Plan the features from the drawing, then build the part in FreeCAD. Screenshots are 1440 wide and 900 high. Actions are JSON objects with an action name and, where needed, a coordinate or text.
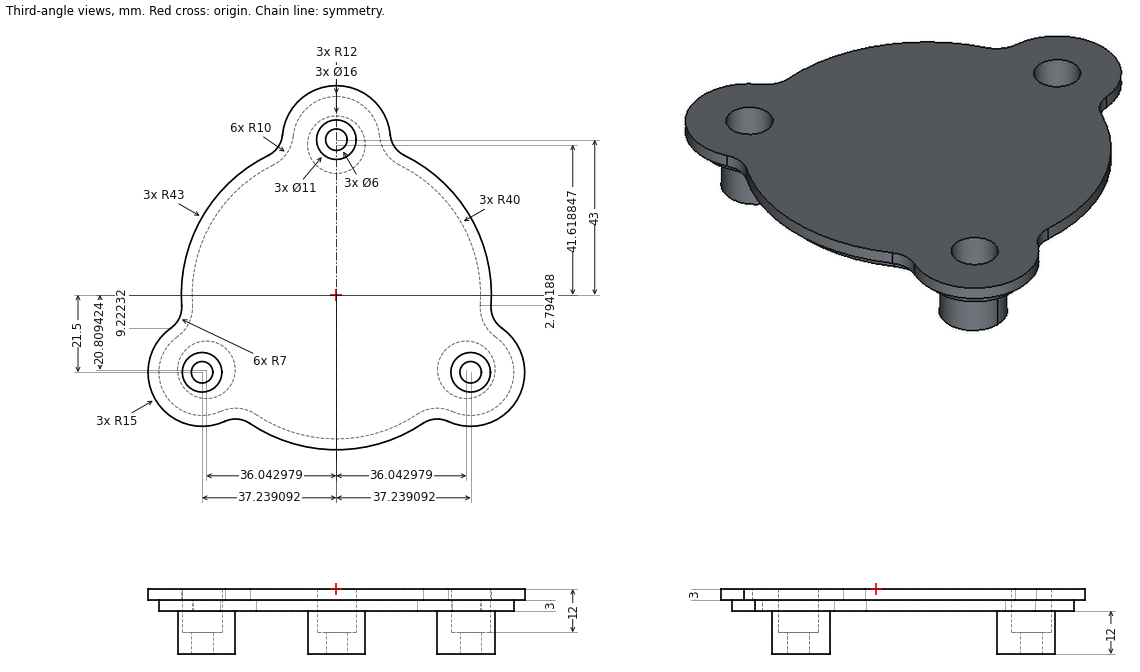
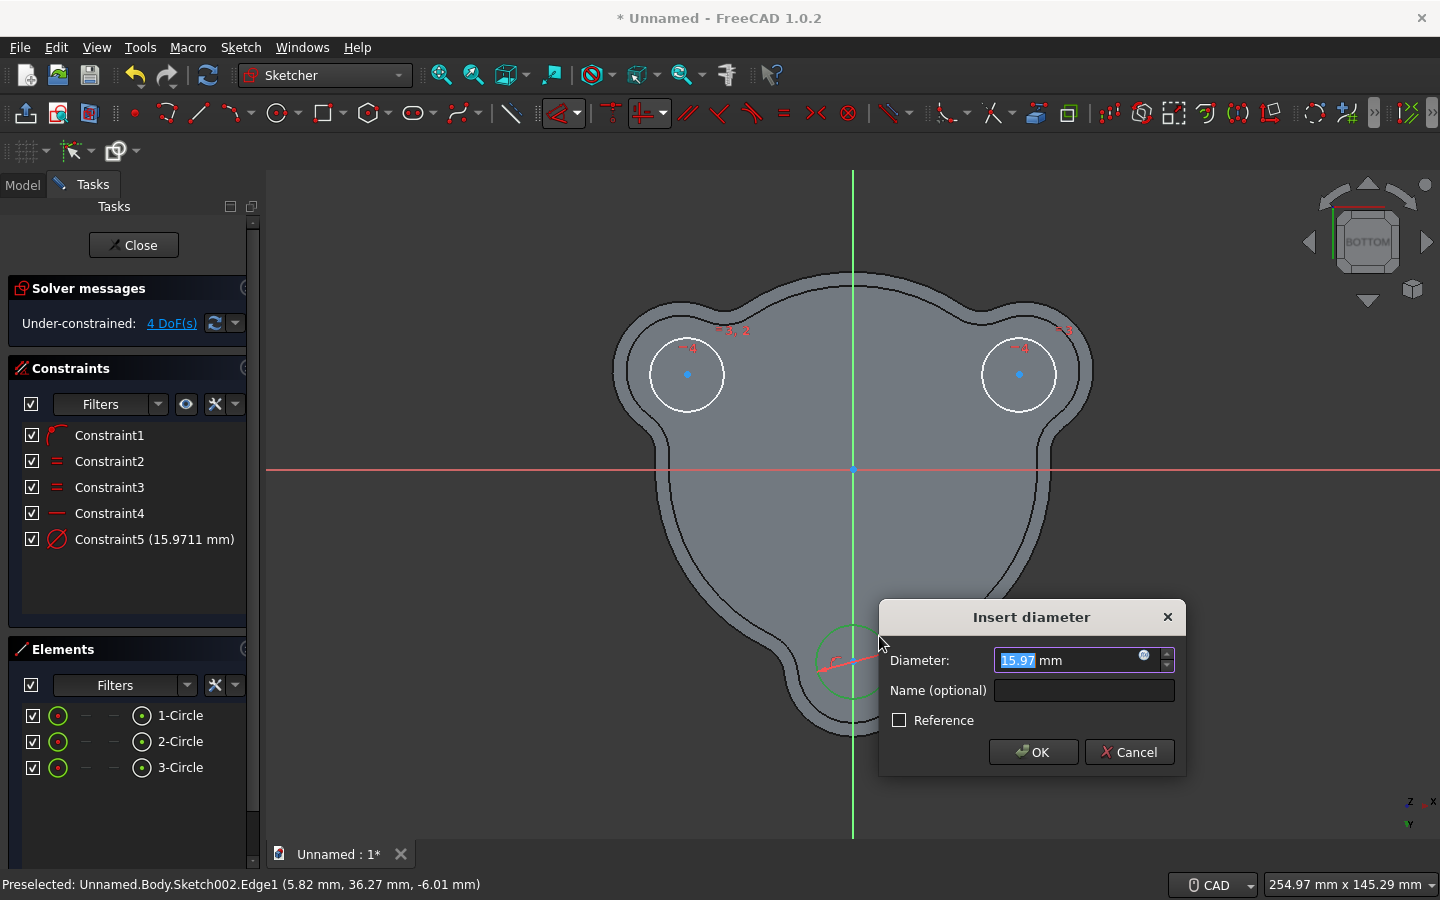
{"action": "type", "text": "16"}
{"action": "key", "text": "Return"}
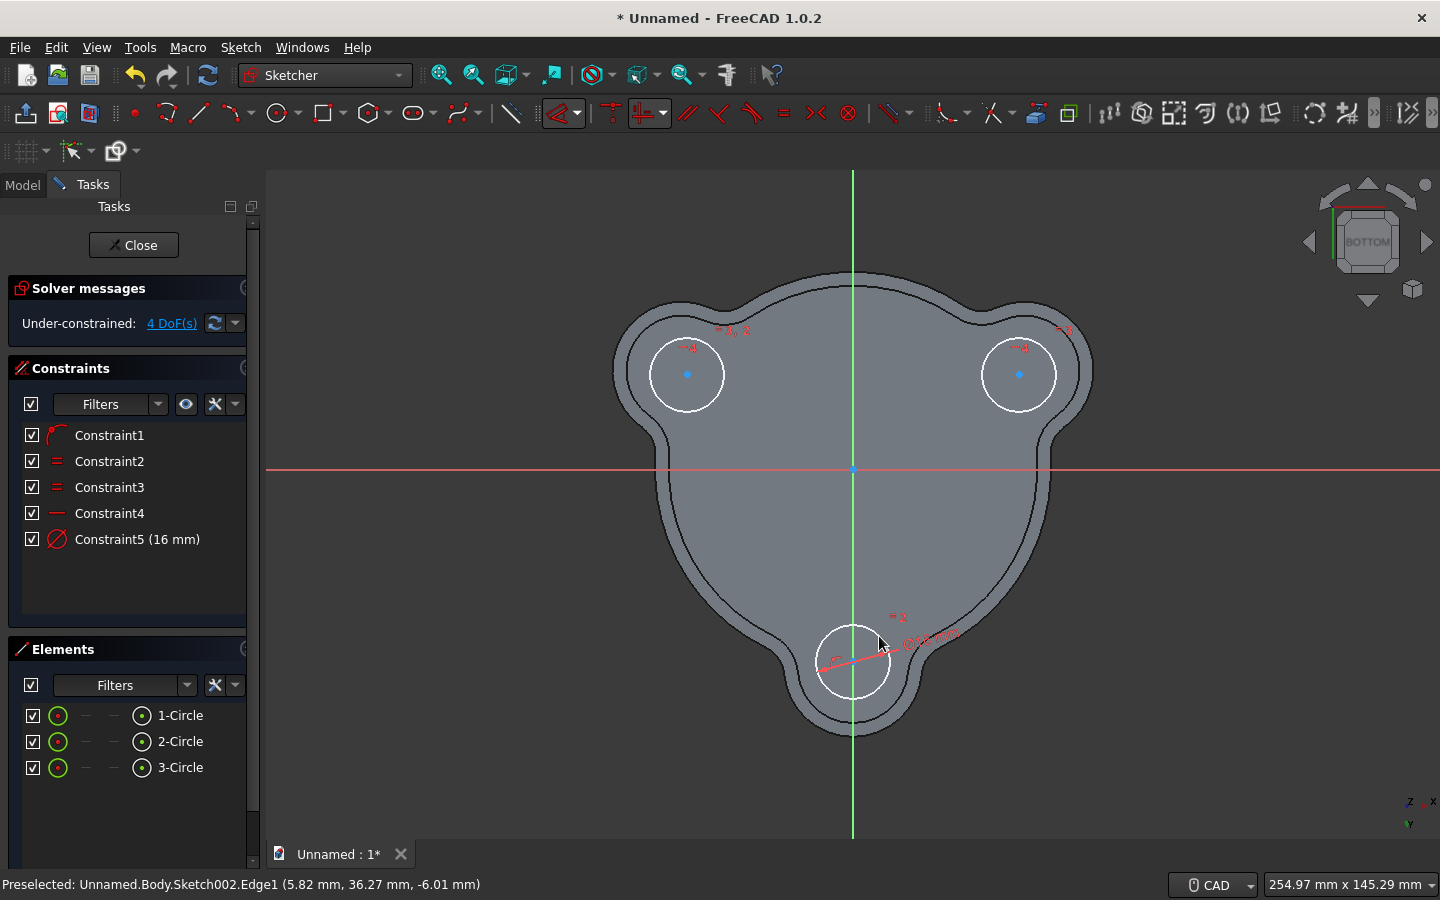
{"action": "left_click", "coordinate": [853, 662]}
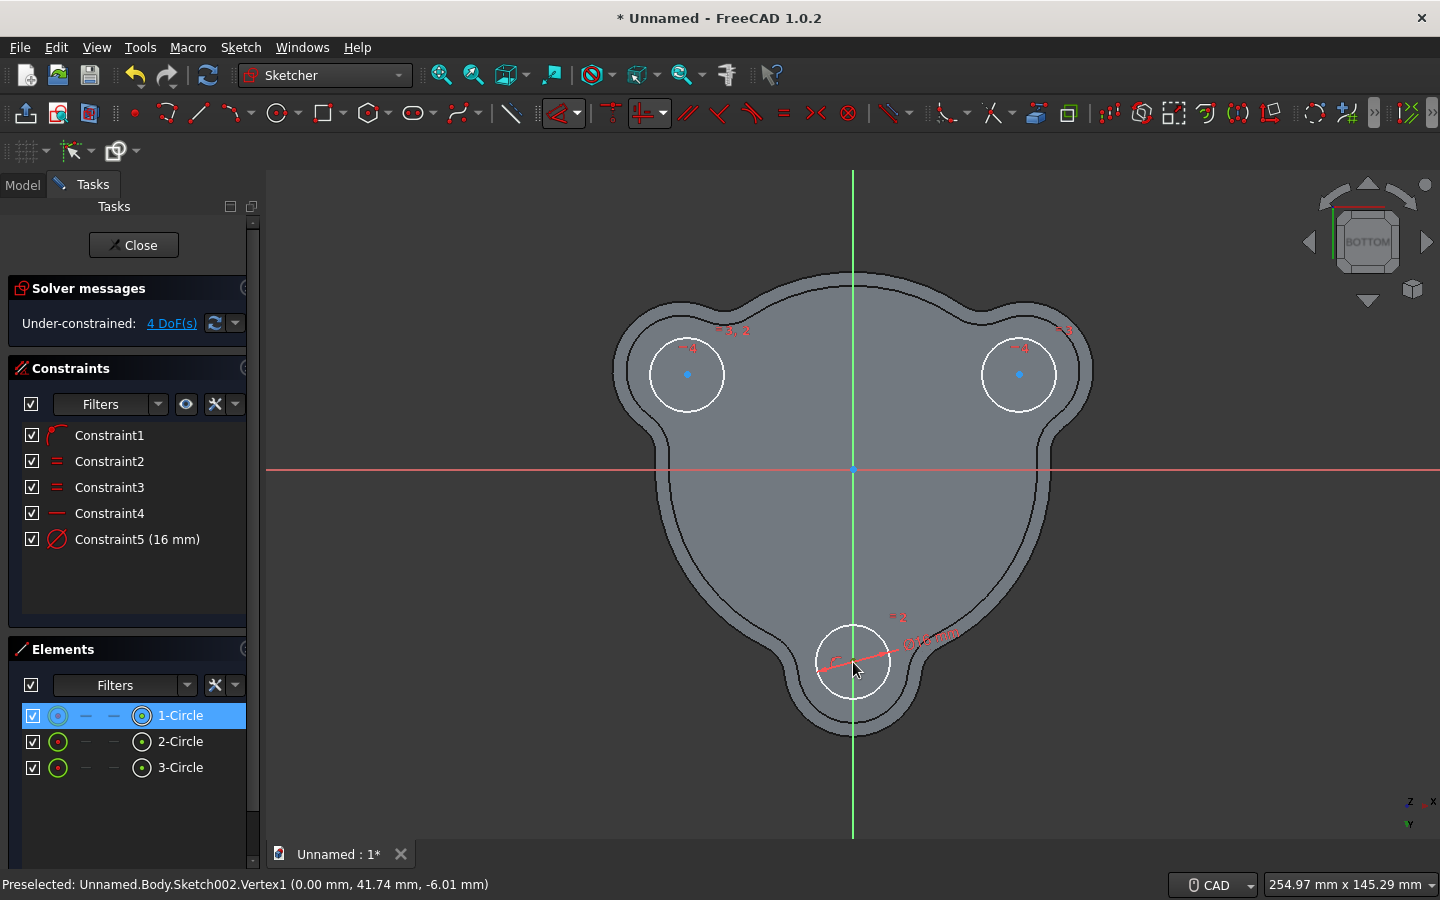
{"action": "left_click", "coordinate": [580, 114]}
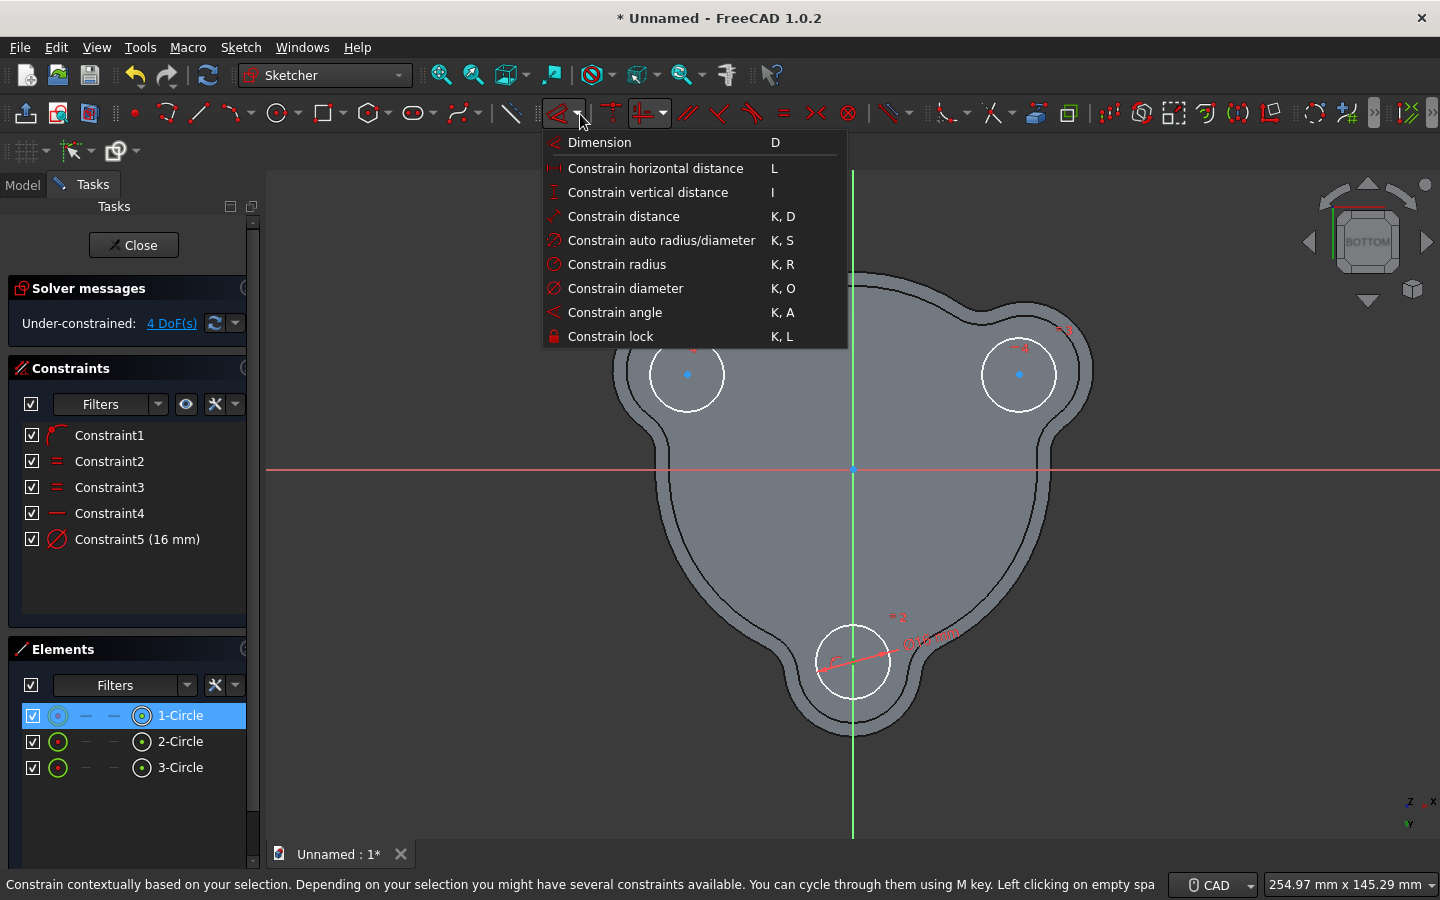
{"action": "left_click", "coordinate": [695, 192]}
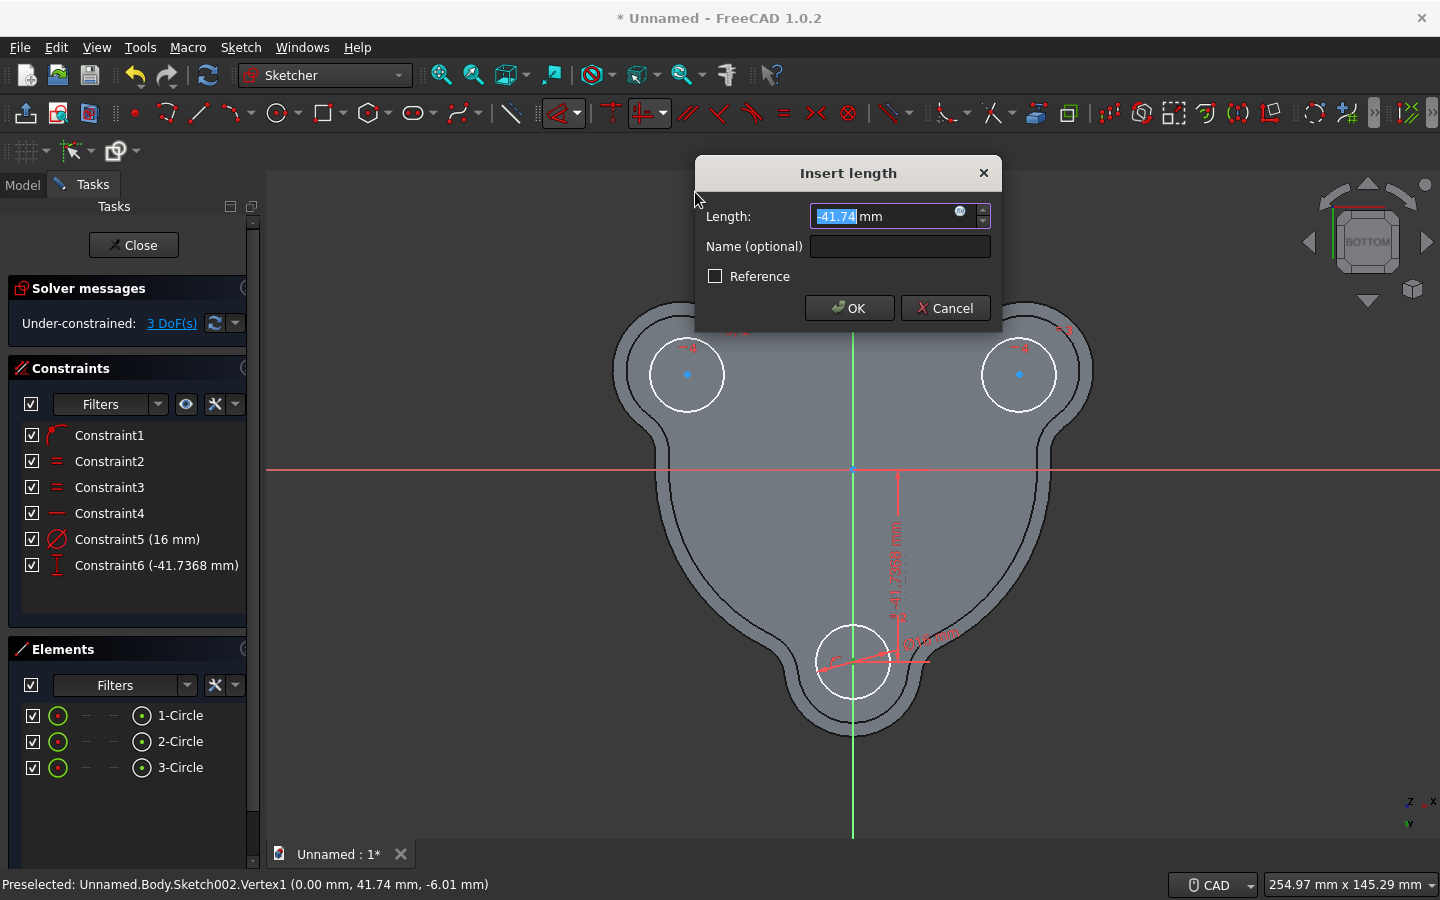
{"action": "type", "text": "-41.618847"}
{"action": "key", "text": "Return"}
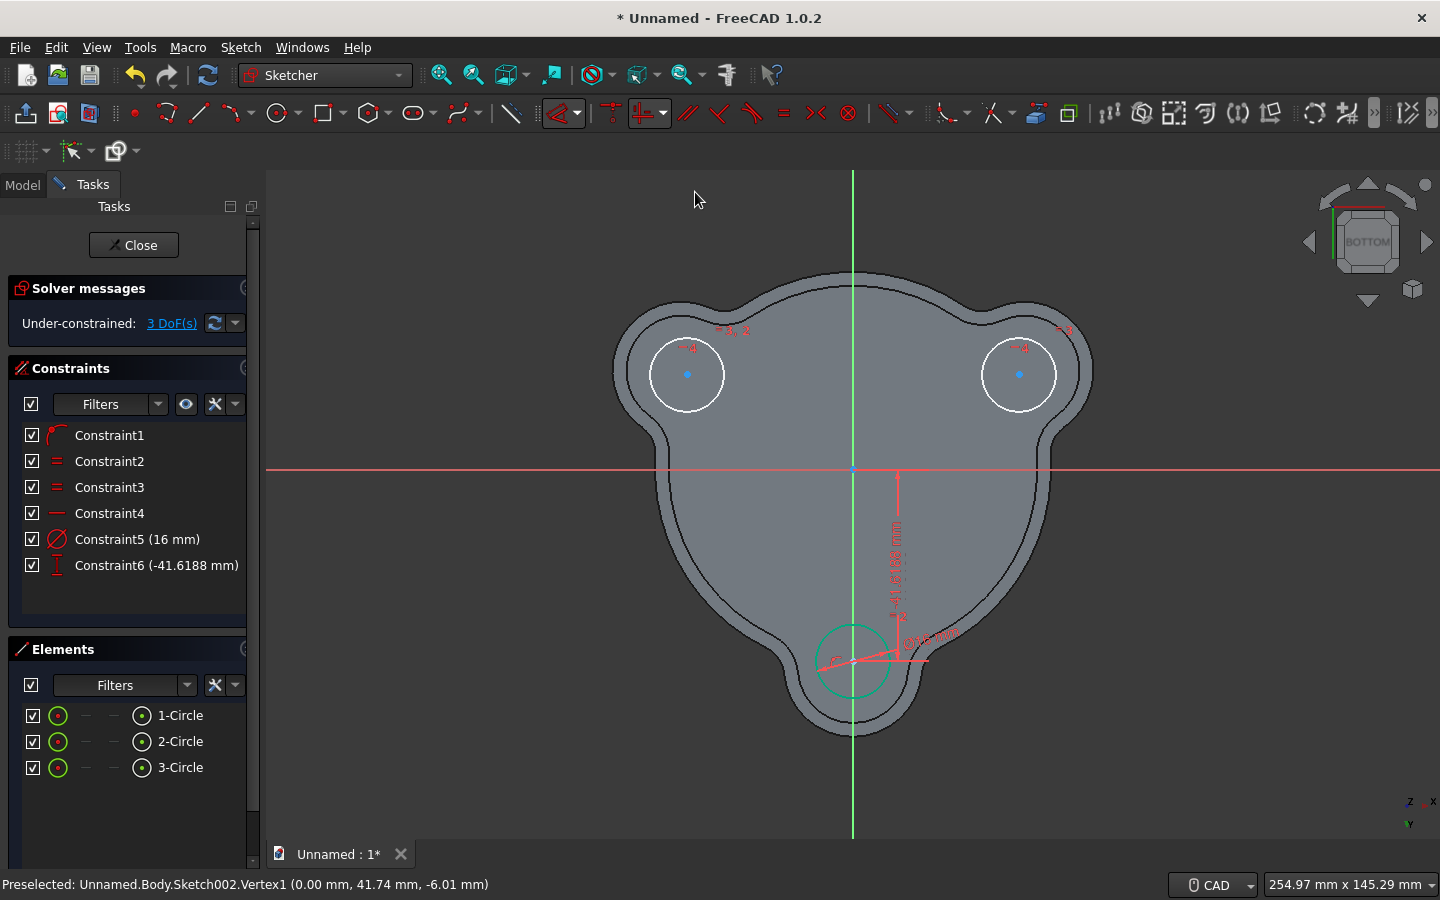
{"action": "left_click", "coordinate": [687, 375]}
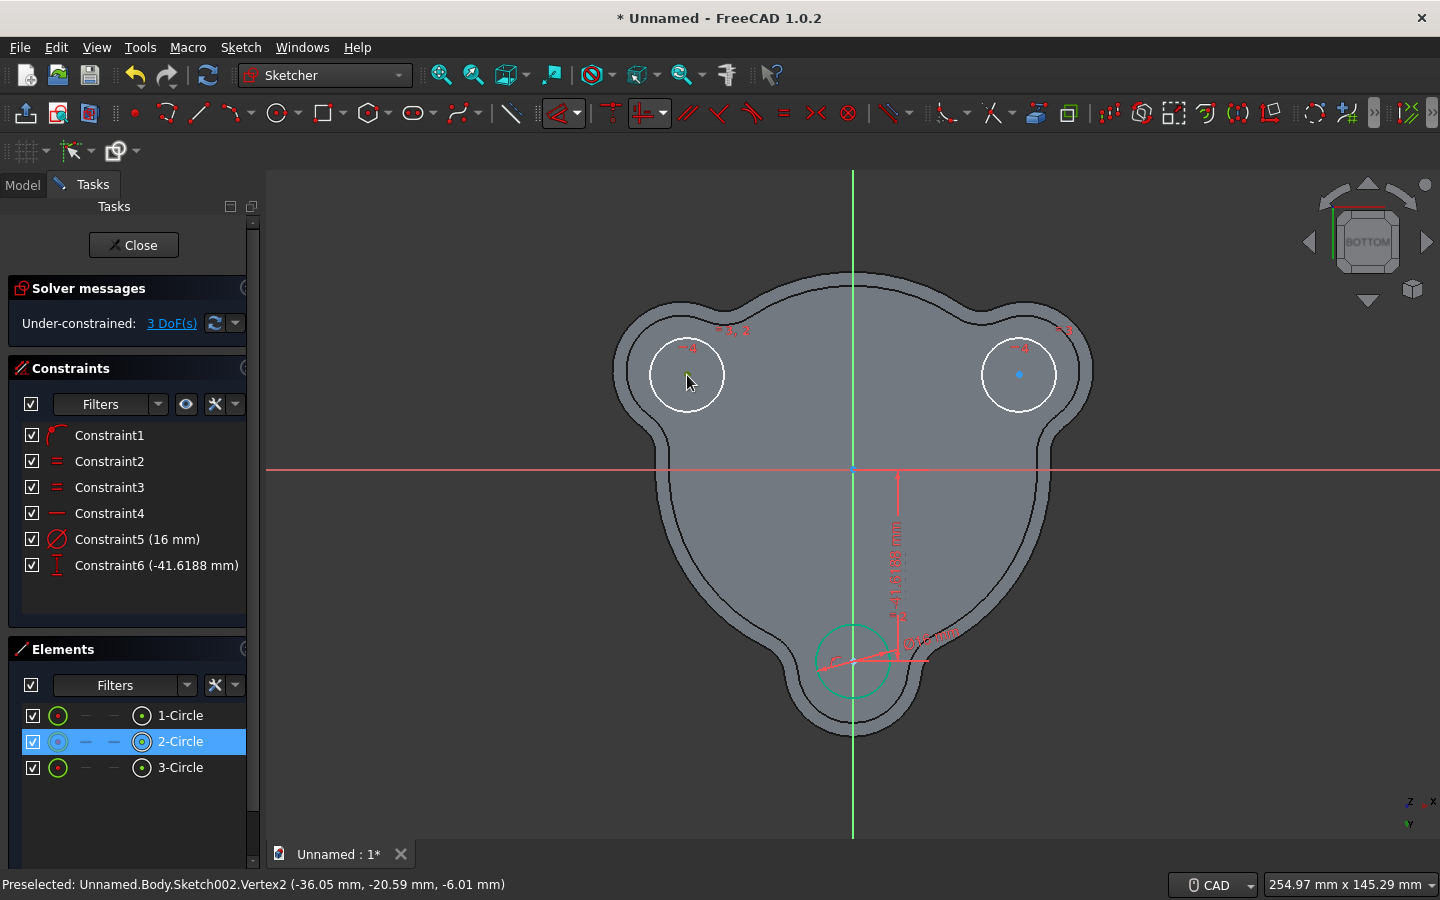
{"action": "key", "text": "l"}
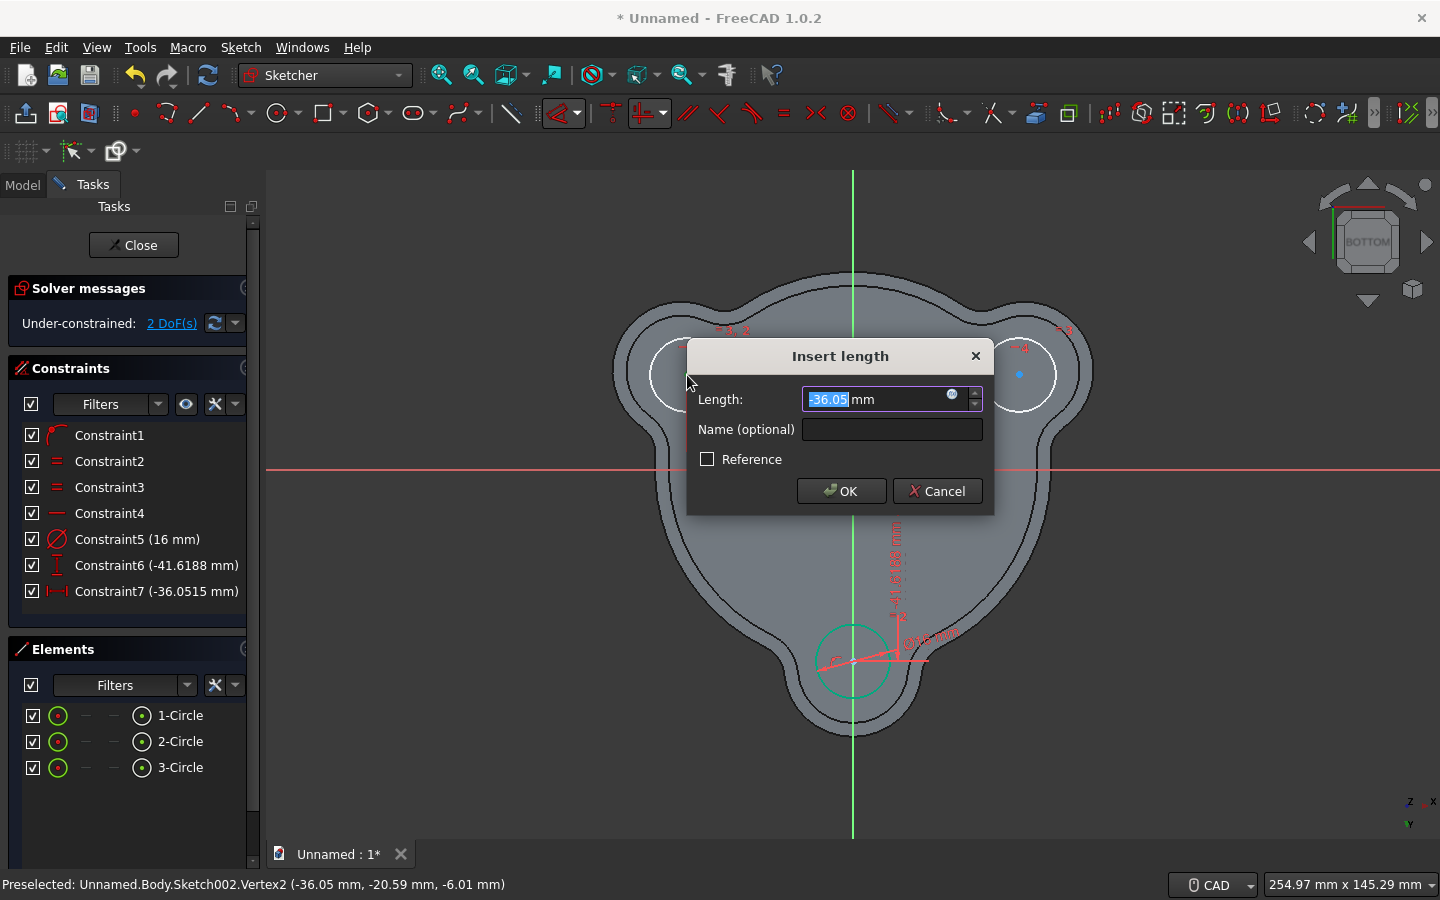
{"action": "type", "text": "-36.042979"}
{"action": "key", "text": "Return"}